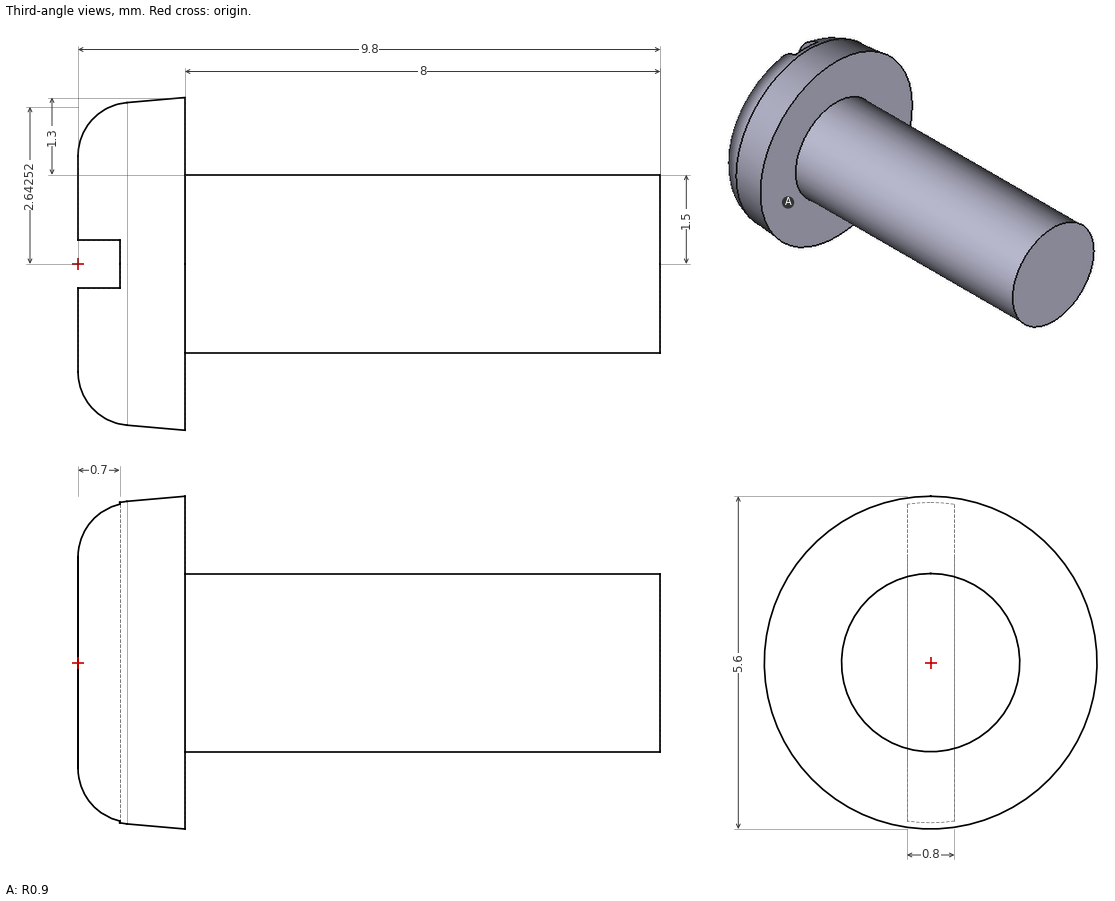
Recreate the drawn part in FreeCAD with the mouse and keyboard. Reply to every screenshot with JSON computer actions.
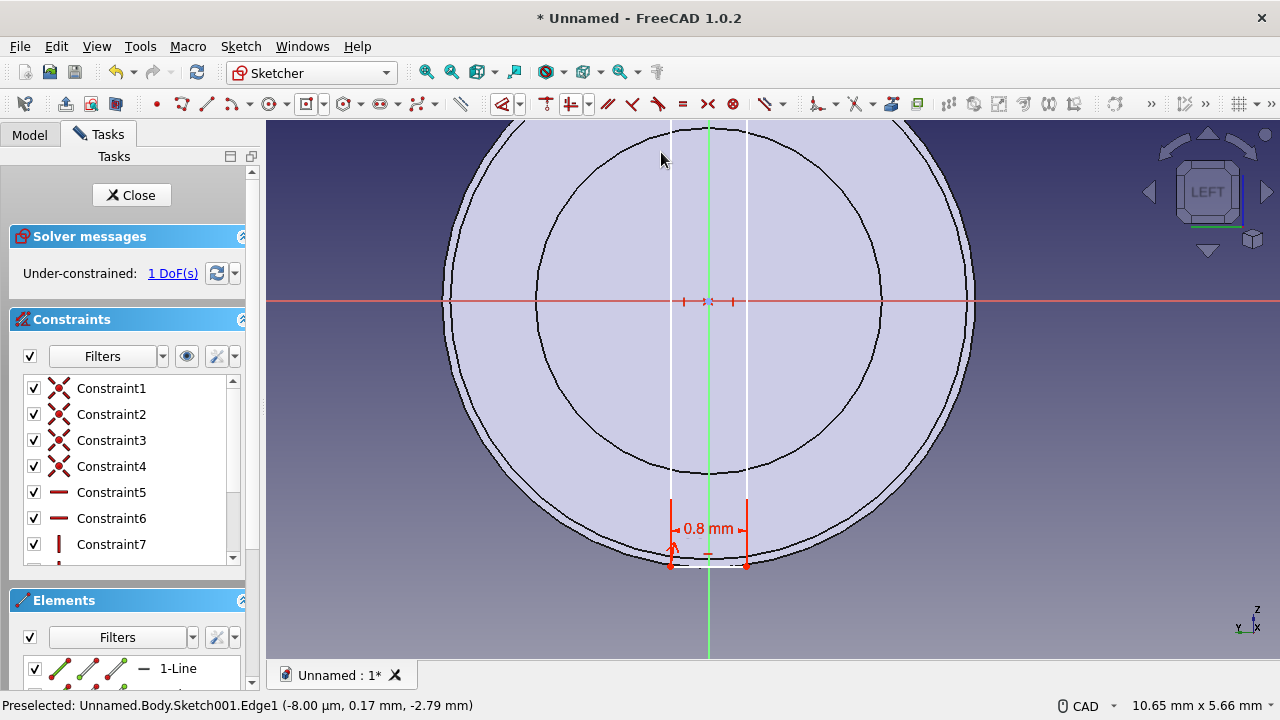
{"action": "left_click", "coordinate": [747, 407]}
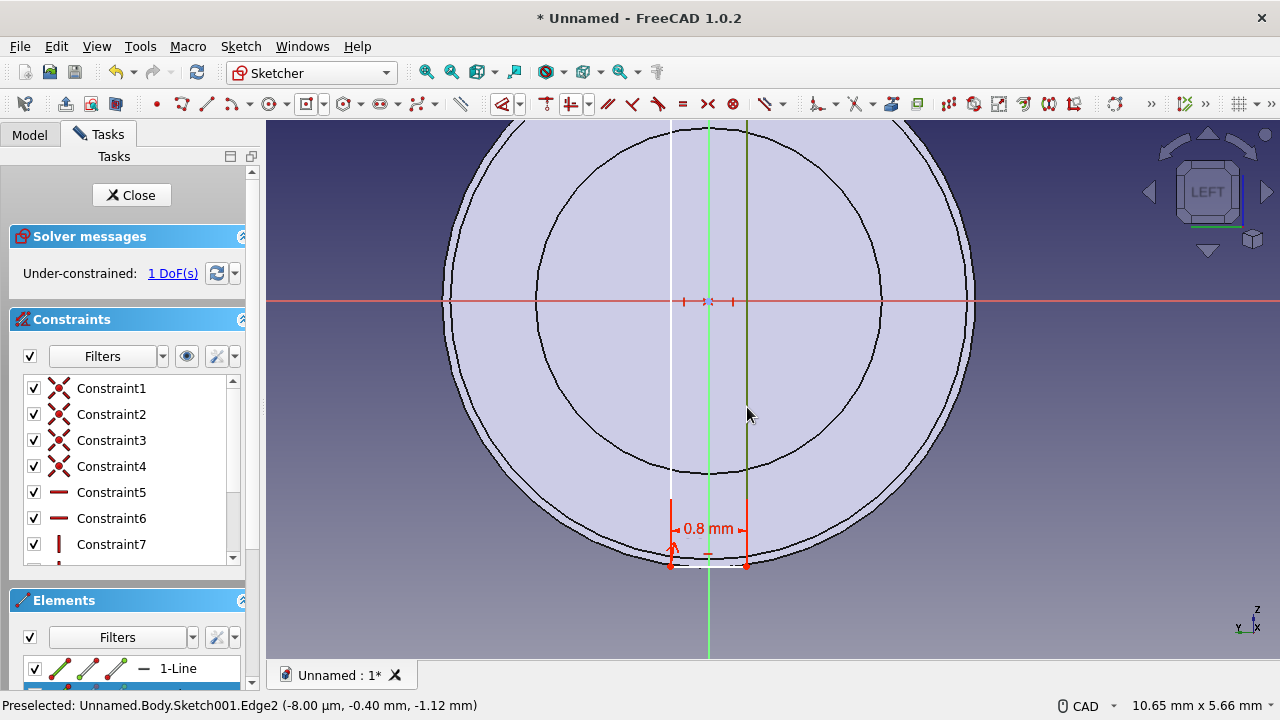
{"action": "left_click", "coordinate": [520, 104]}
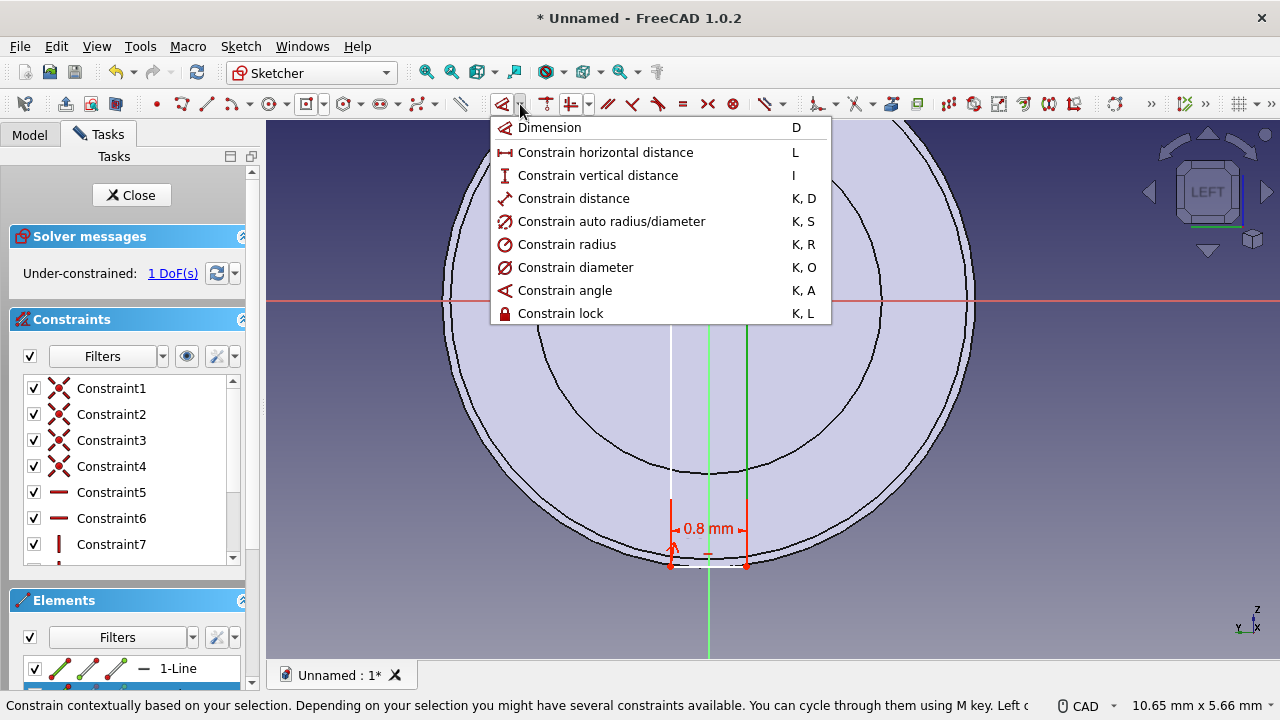
{"action": "left_click", "coordinate": [661, 176]}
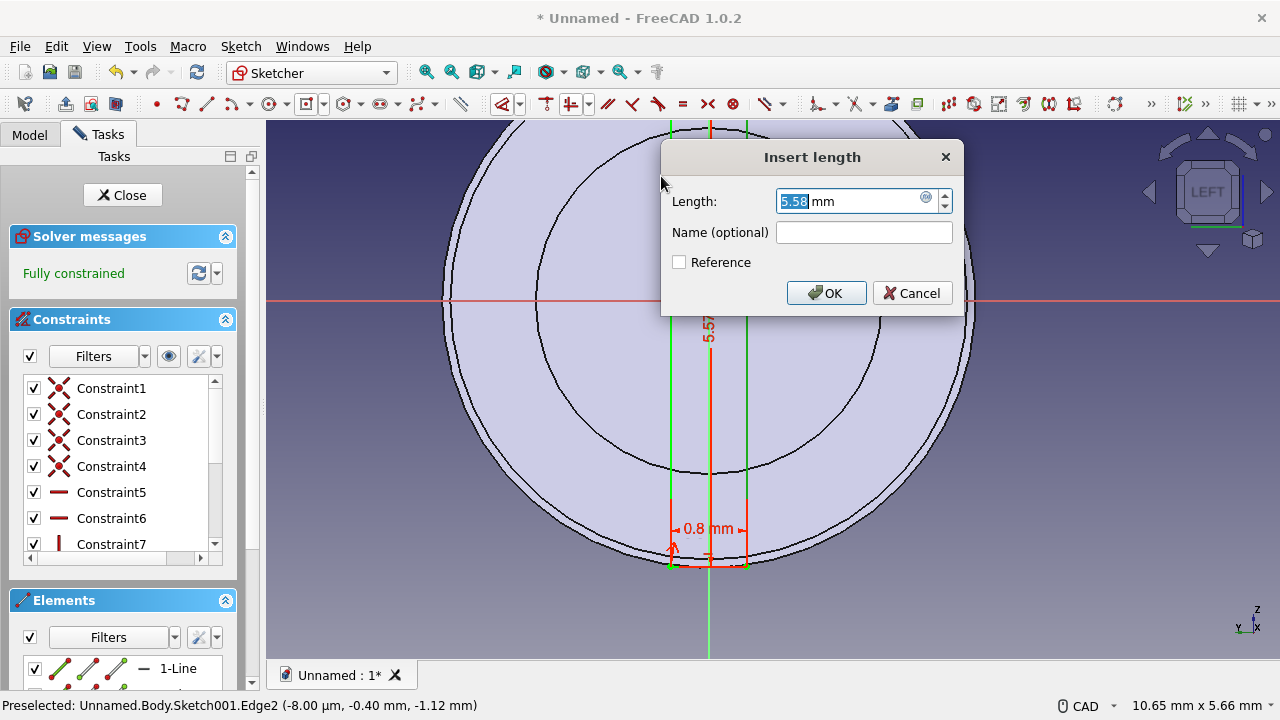
{"action": "type", "text": "5.6"}
{"action": "key", "text": "Return"}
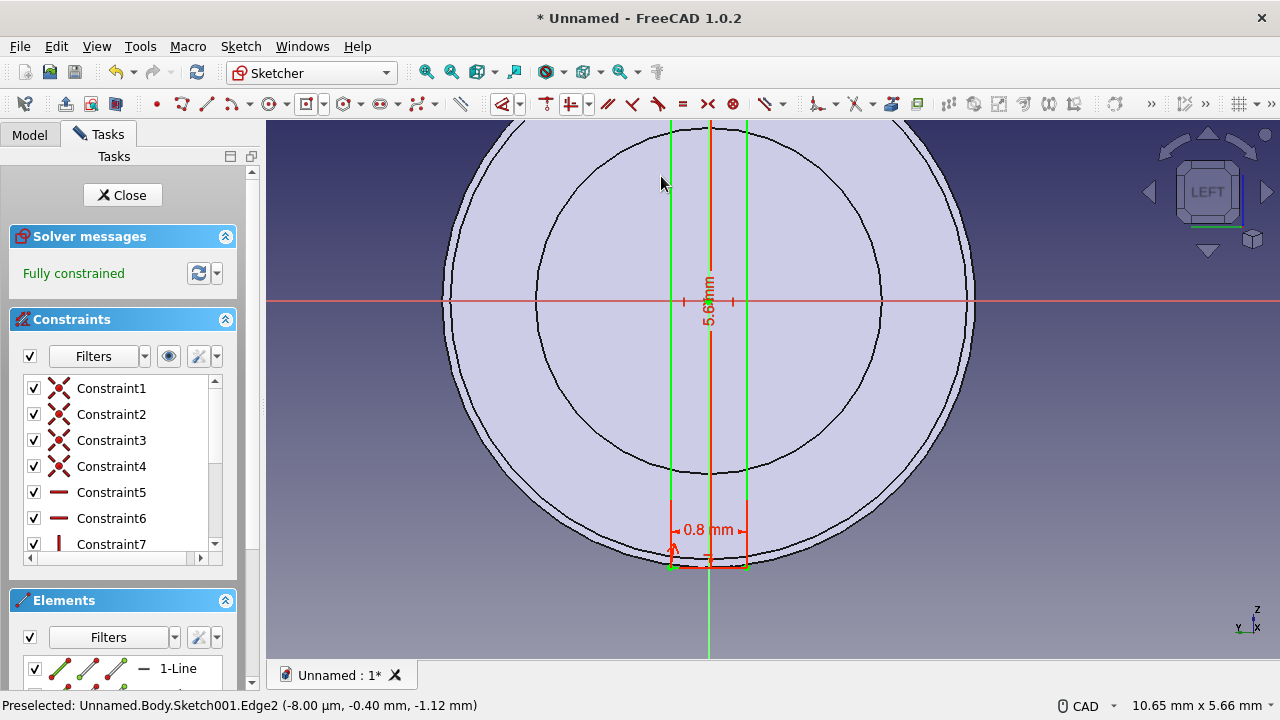
{"action": "left_click", "coordinate": [123, 195]}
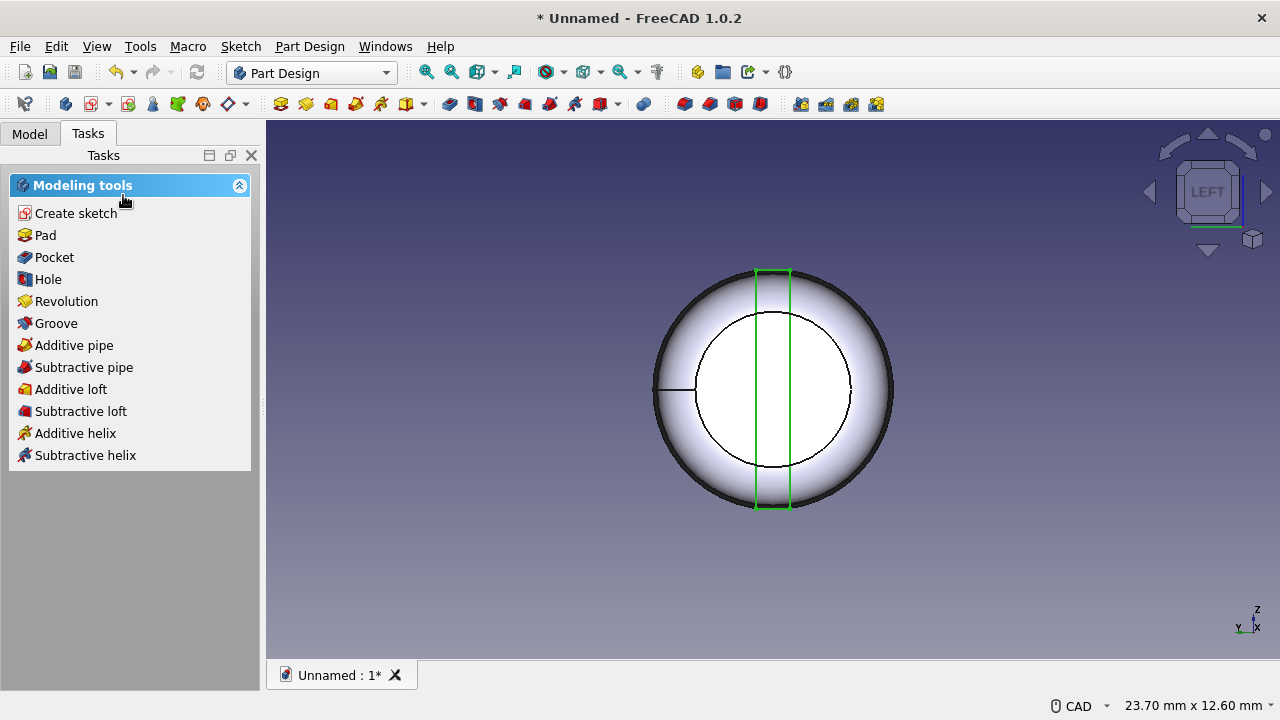
{"action": "left_click", "coordinate": [450, 104]}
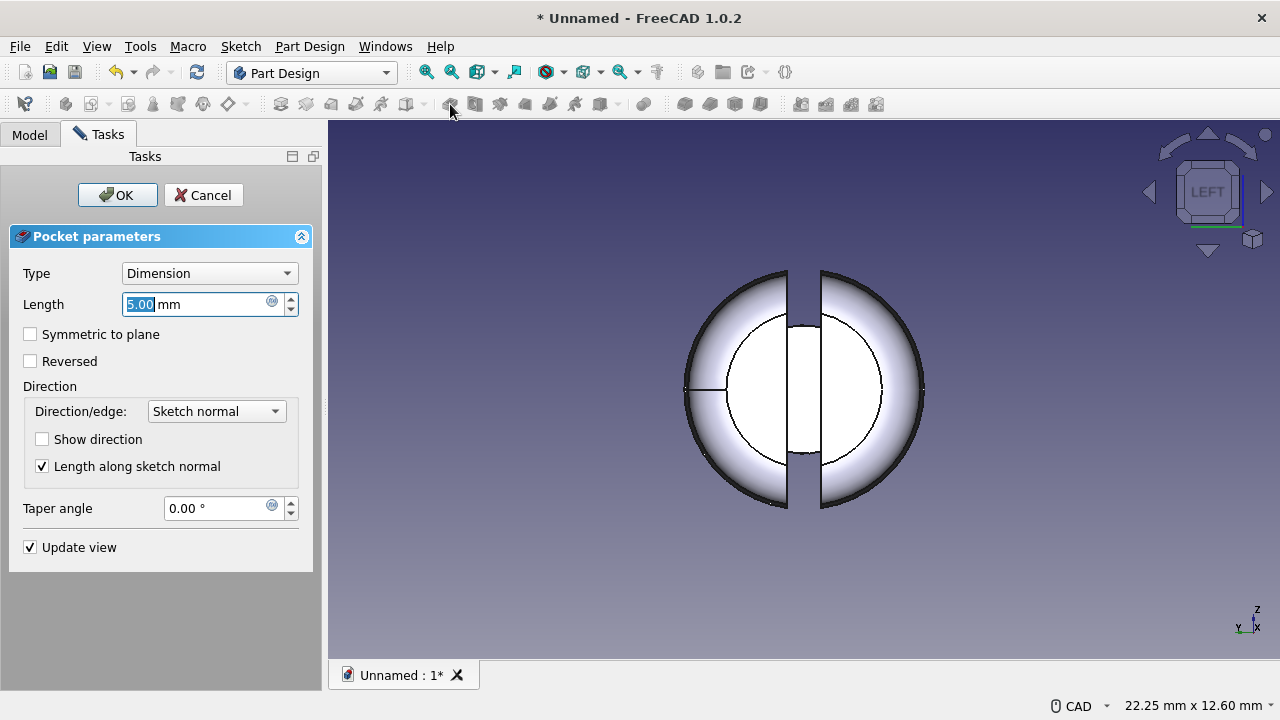
{"action": "type", "text": "0.7"}
{"action": "key", "text": "Tab"}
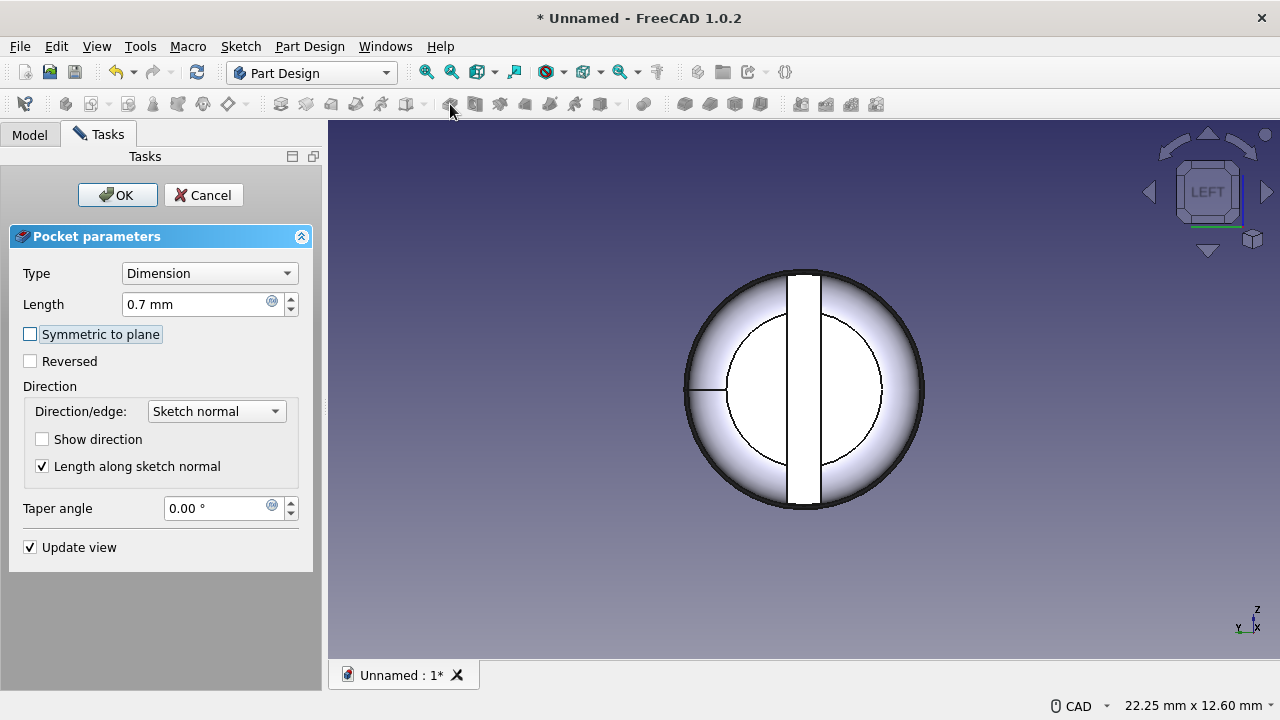
{"action": "left_click", "coordinate": [118, 195]}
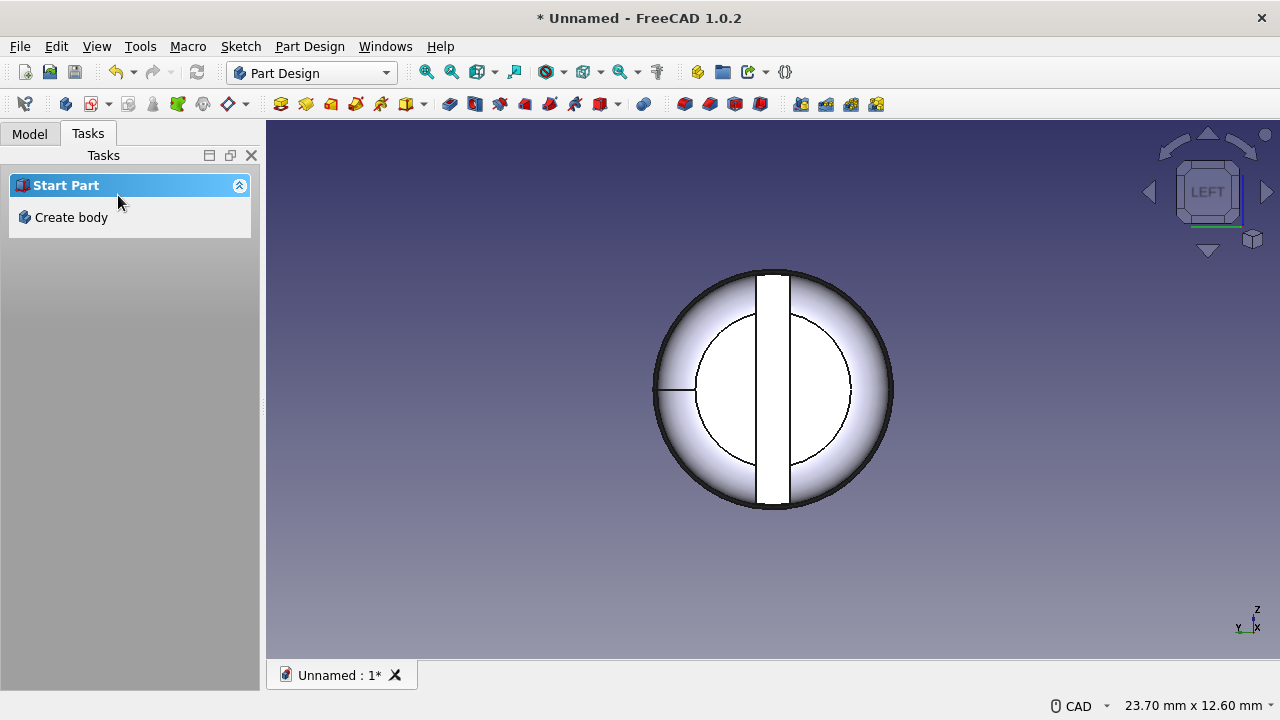
{"action": "key", "text": "0"}